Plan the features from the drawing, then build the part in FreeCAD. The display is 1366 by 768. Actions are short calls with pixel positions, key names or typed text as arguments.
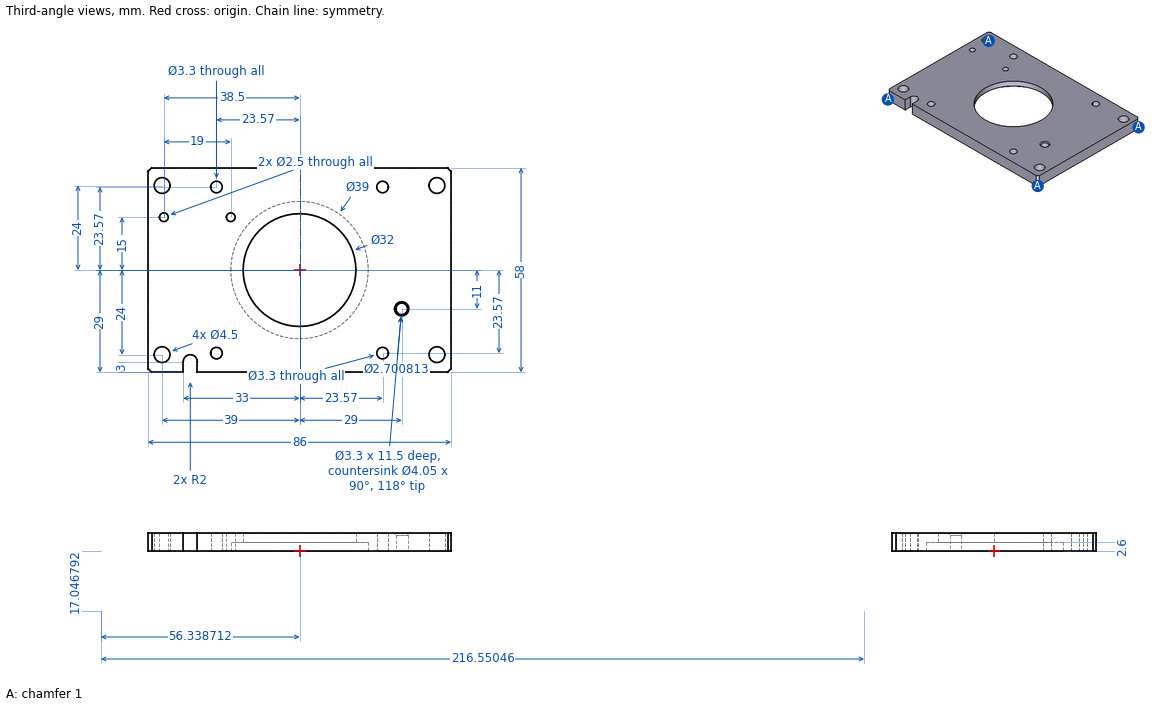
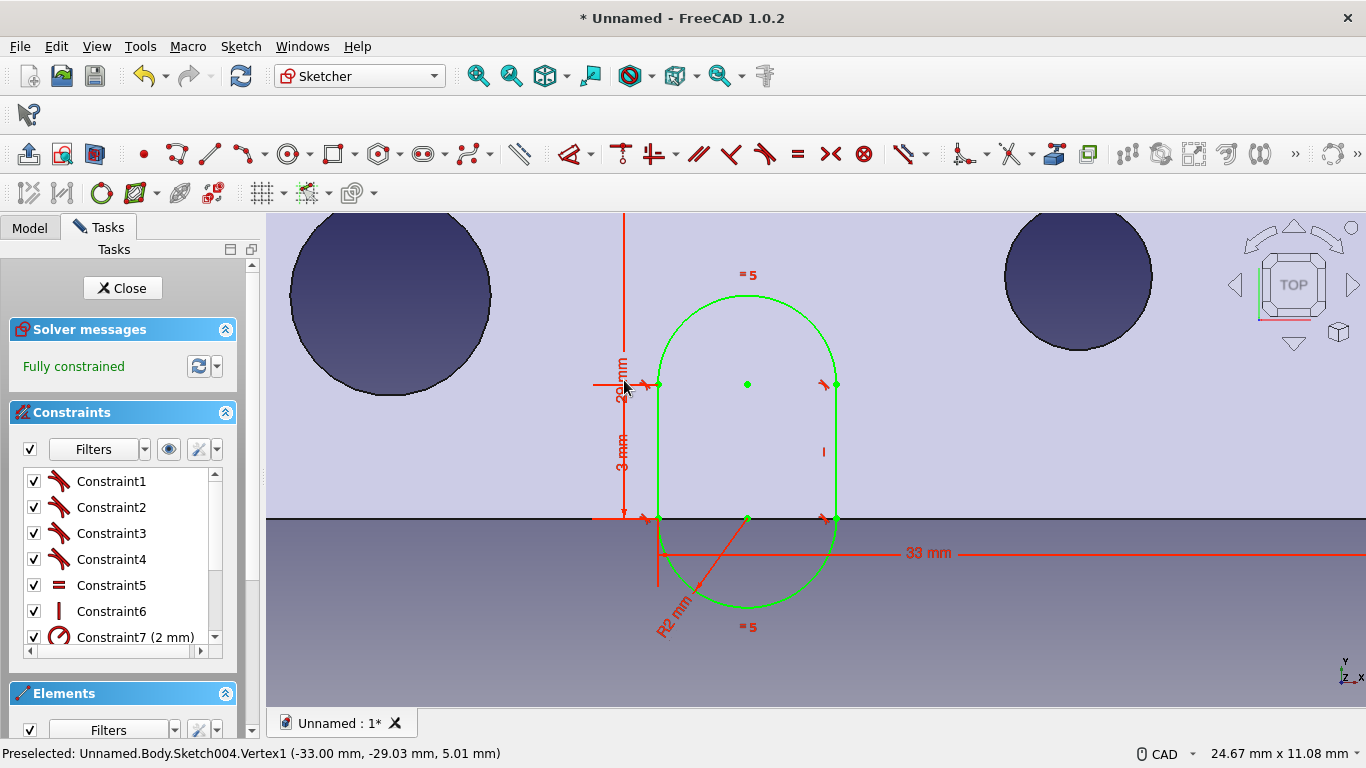
click(123, 288)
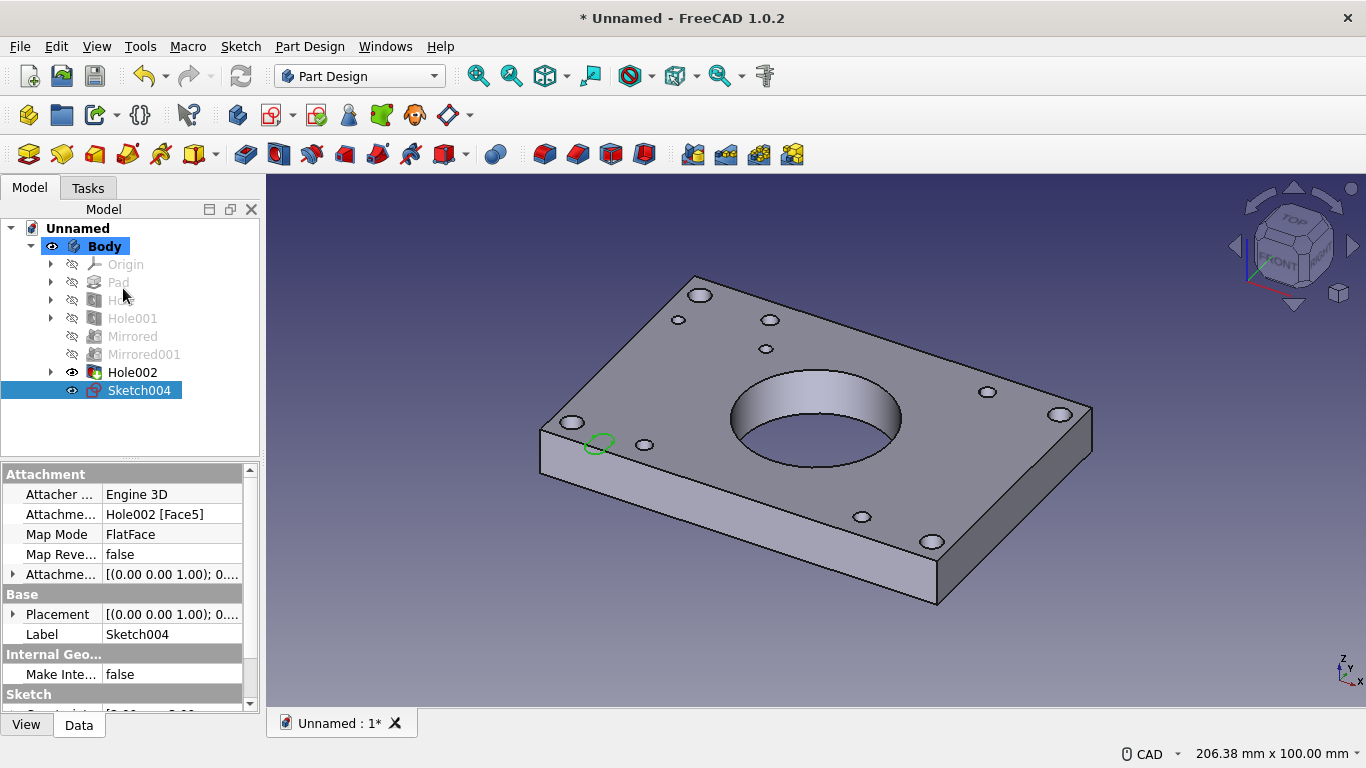
click(246, 154)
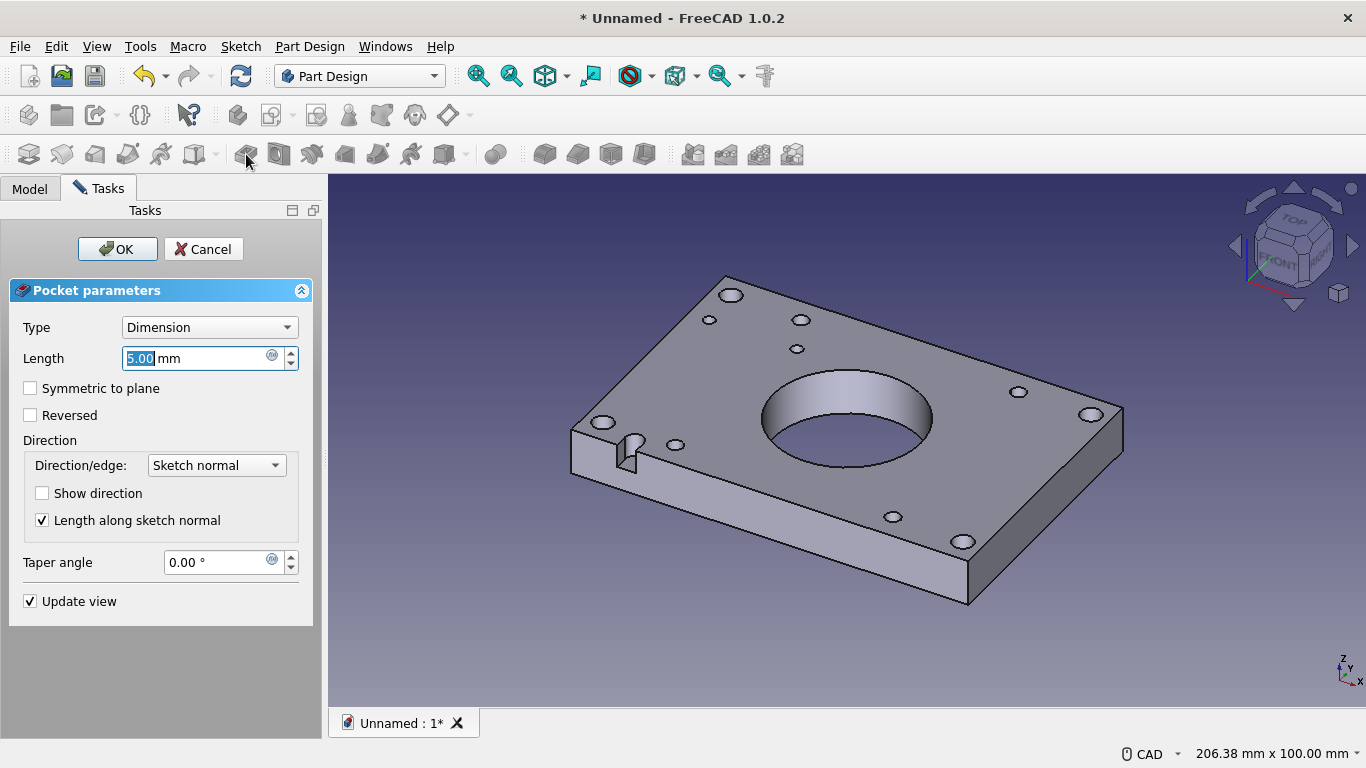
click(210, 328)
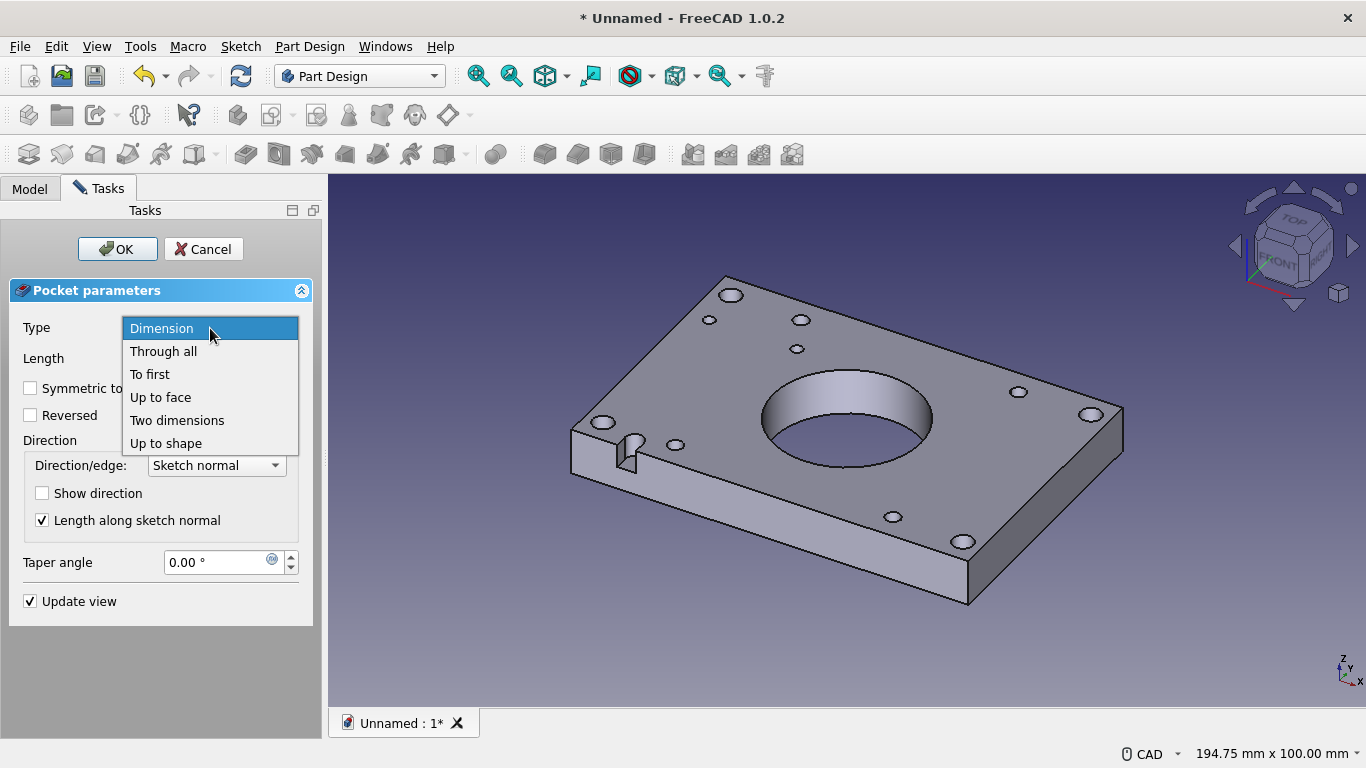
click(208, 352)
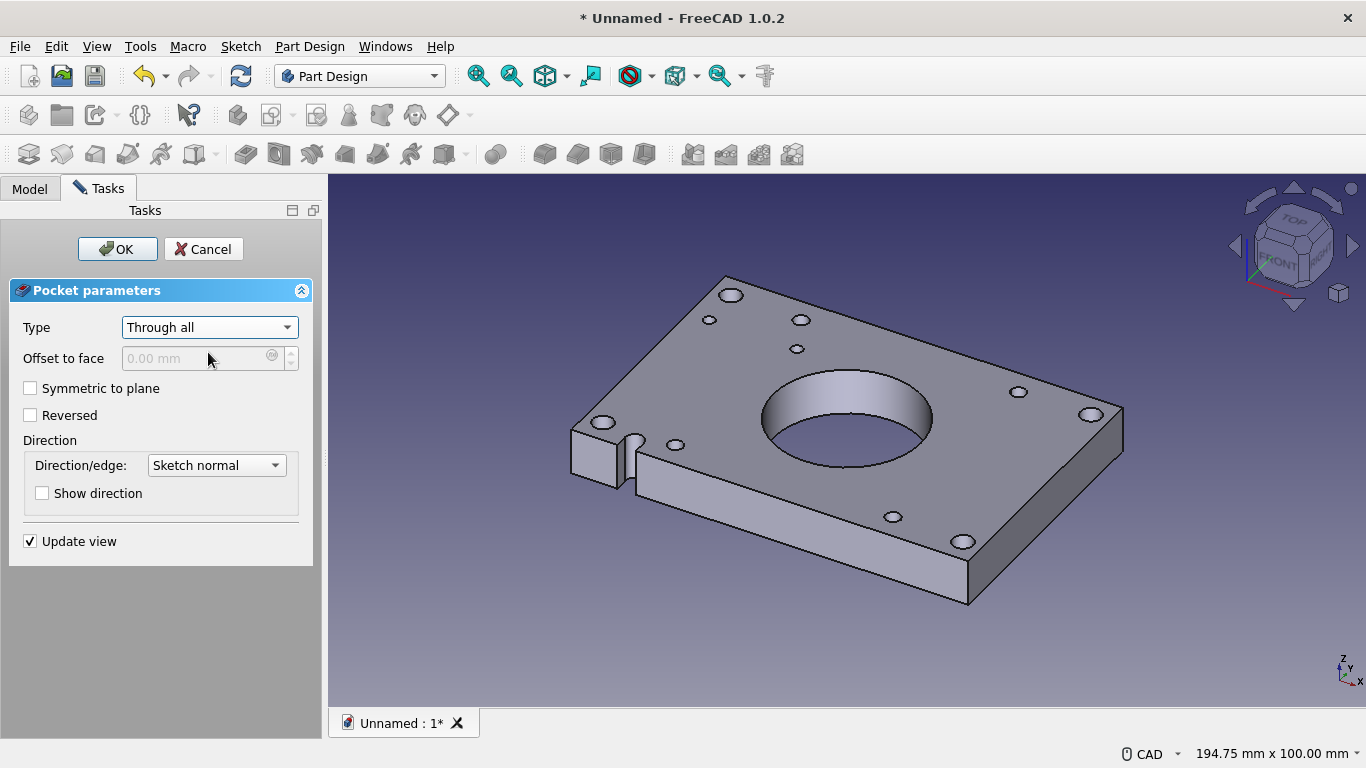
click(118, 249)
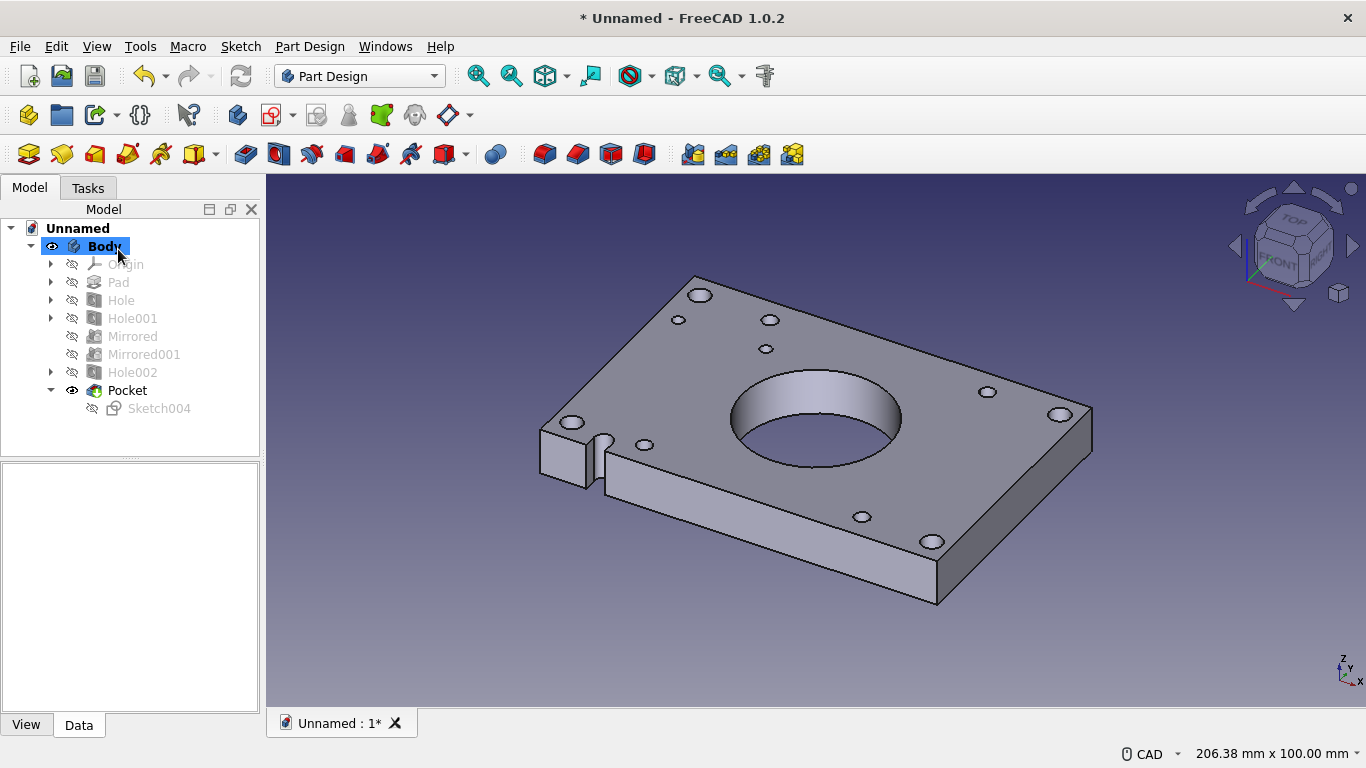
click(937, 582)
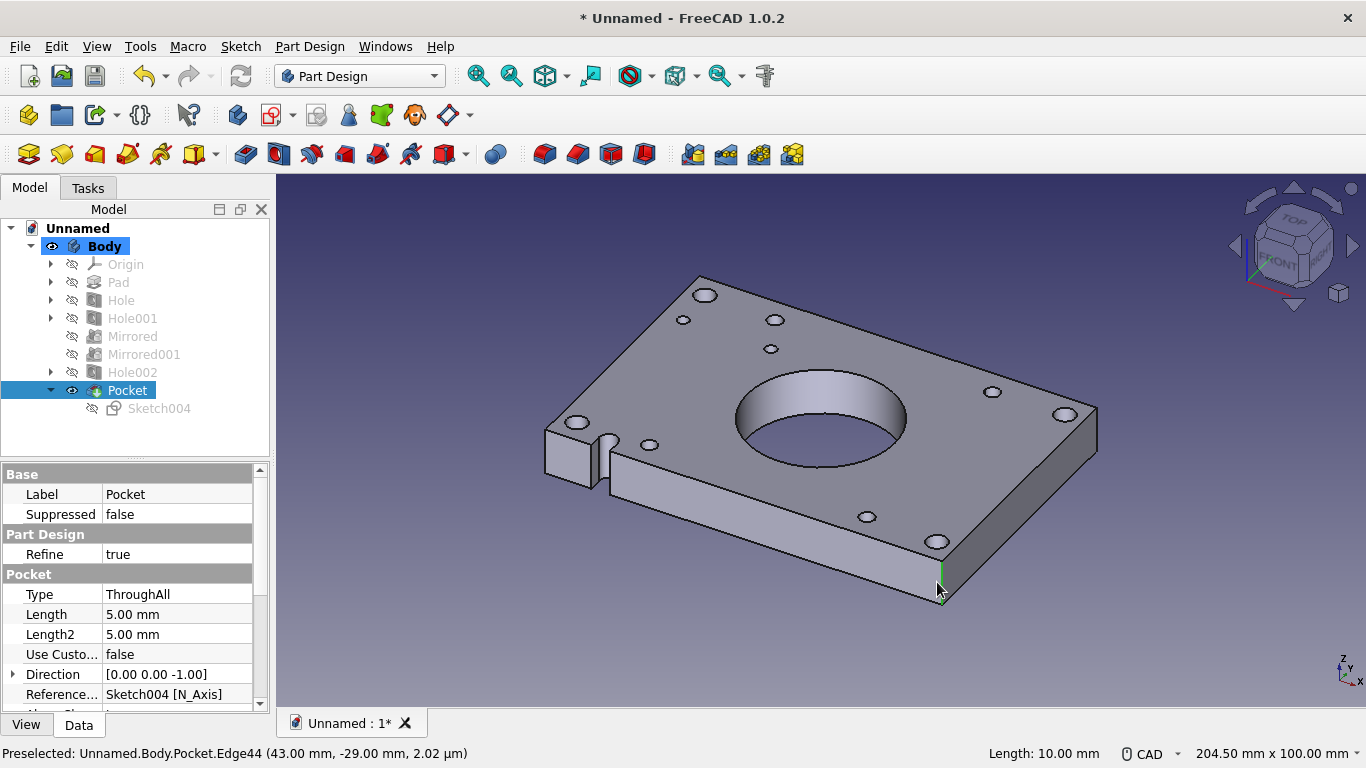
key(0)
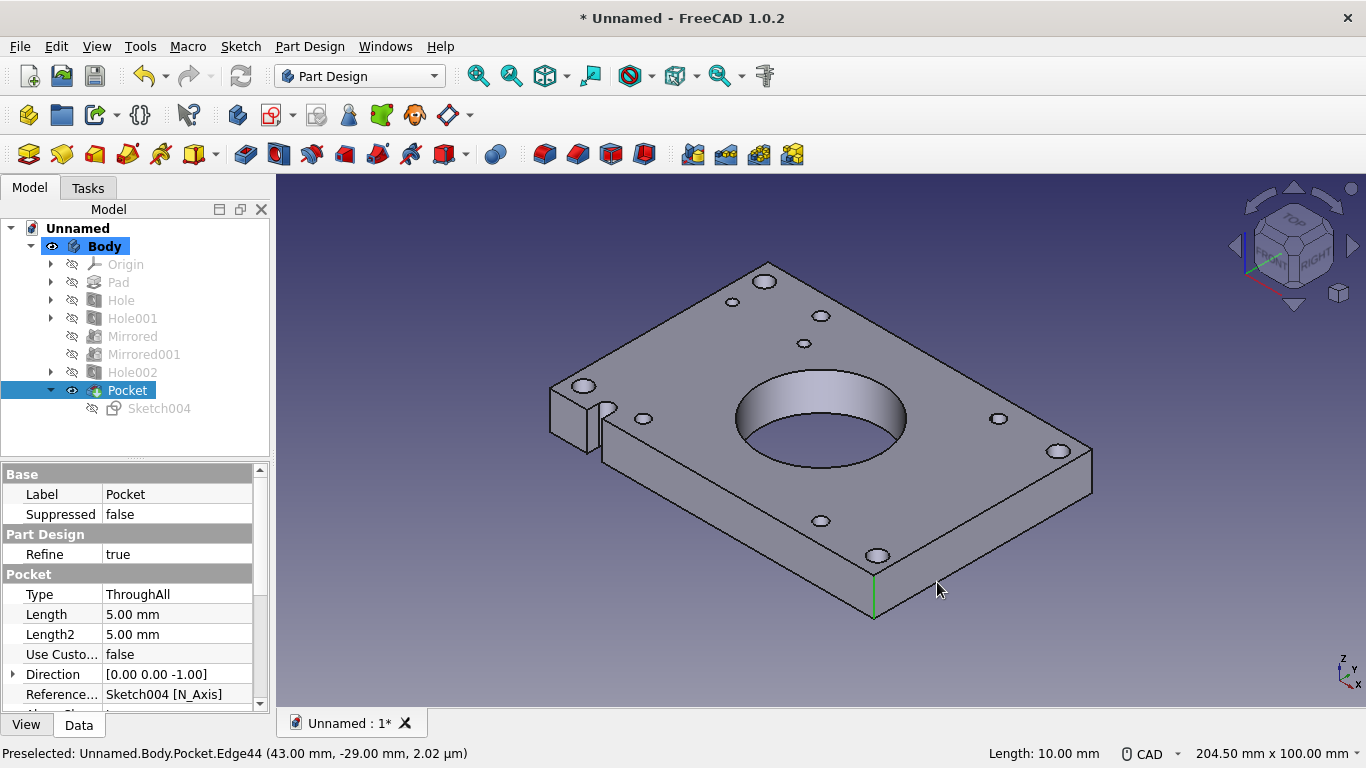
key(2)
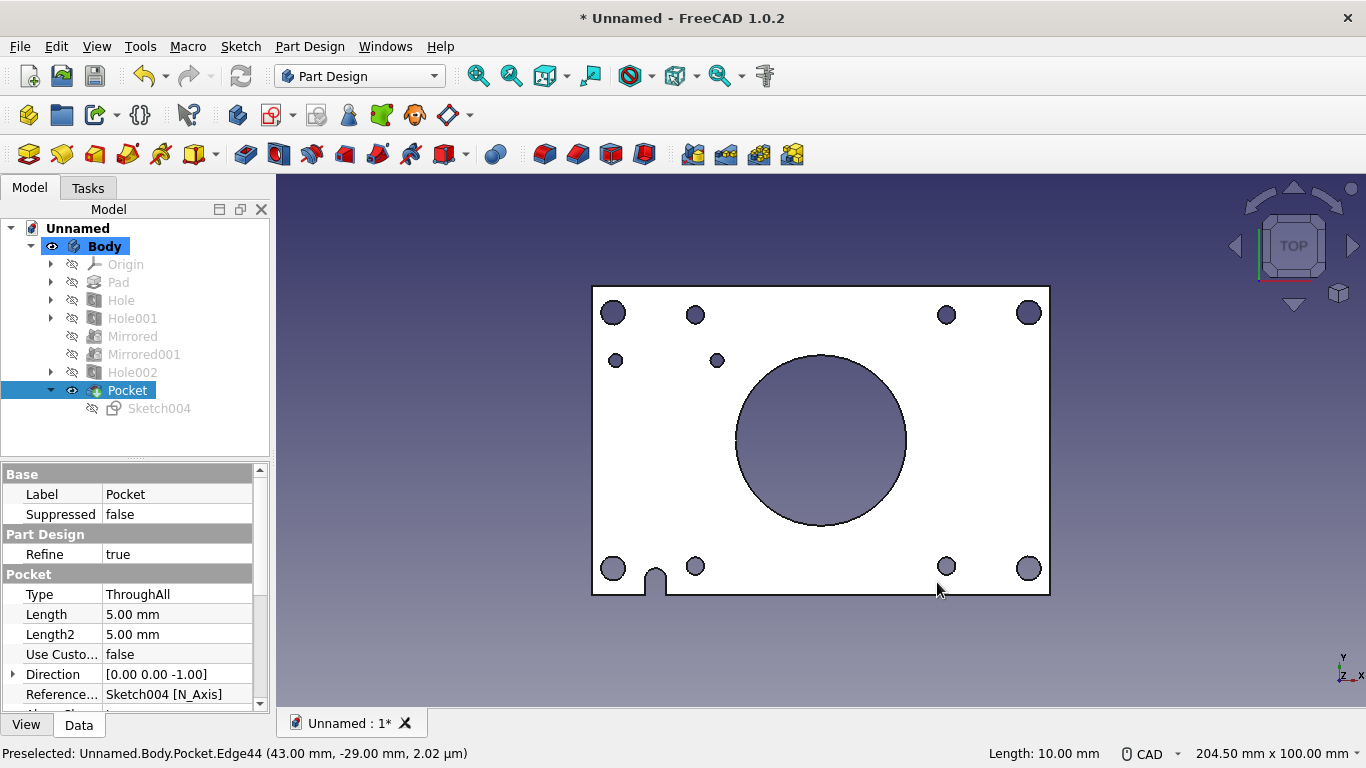
key(1)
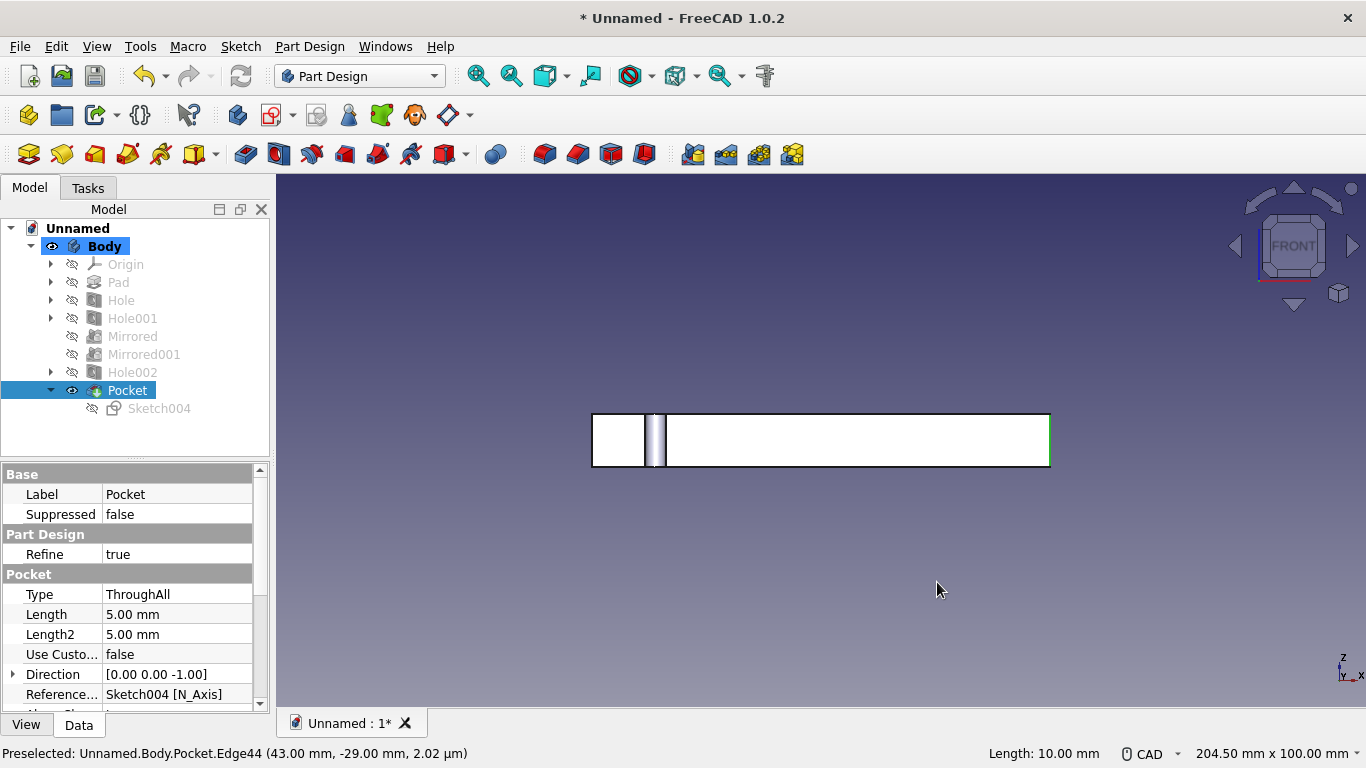
key(v)
key(f)